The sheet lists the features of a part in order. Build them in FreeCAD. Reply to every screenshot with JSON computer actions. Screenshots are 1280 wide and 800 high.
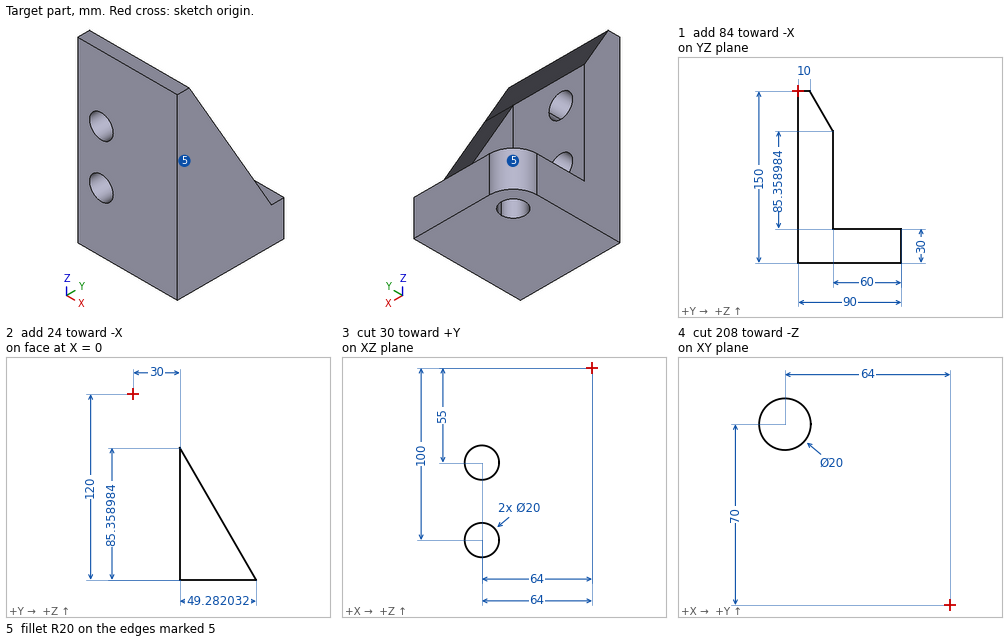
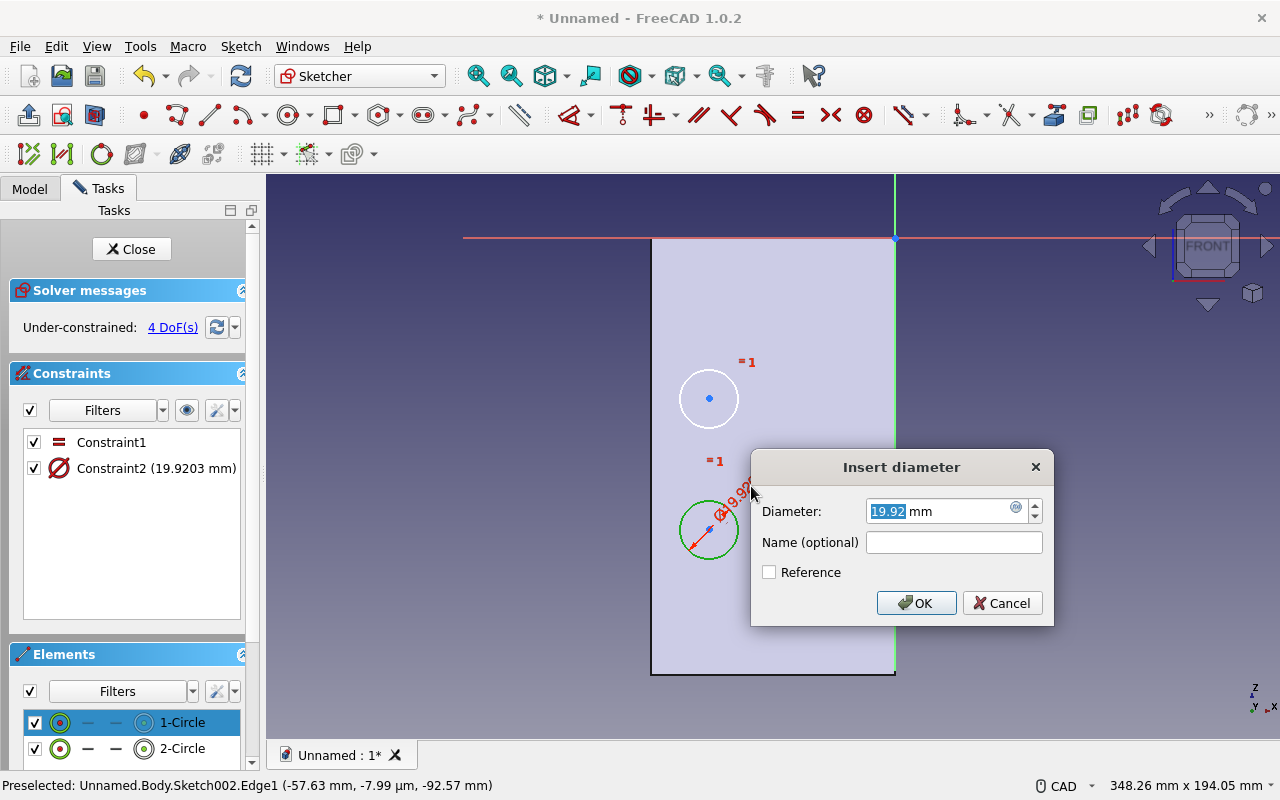
{"action": "type", "text": "20"}
{"action": "key", "text": "Return"}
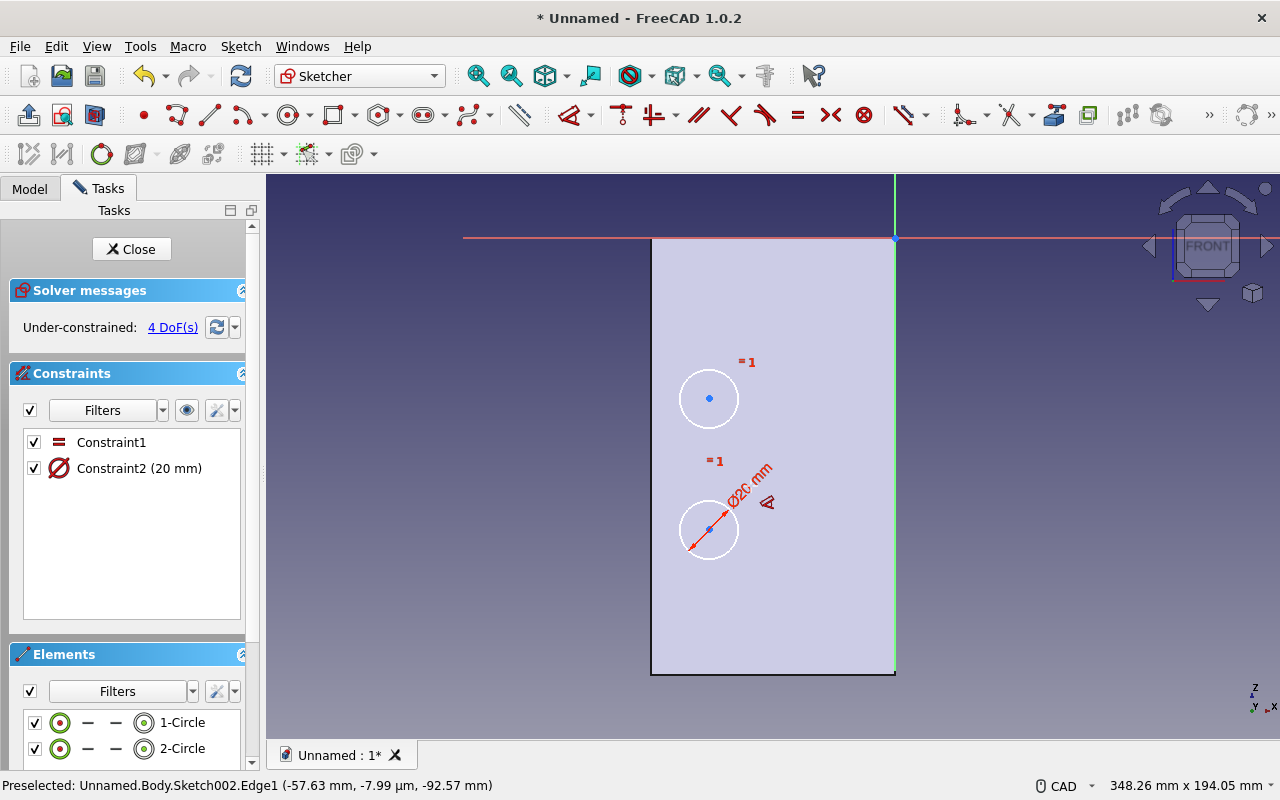
{"action": "left_click", "coordinate": [709, 530]}
{"action": "left_click", "coordinate": [802, 204]}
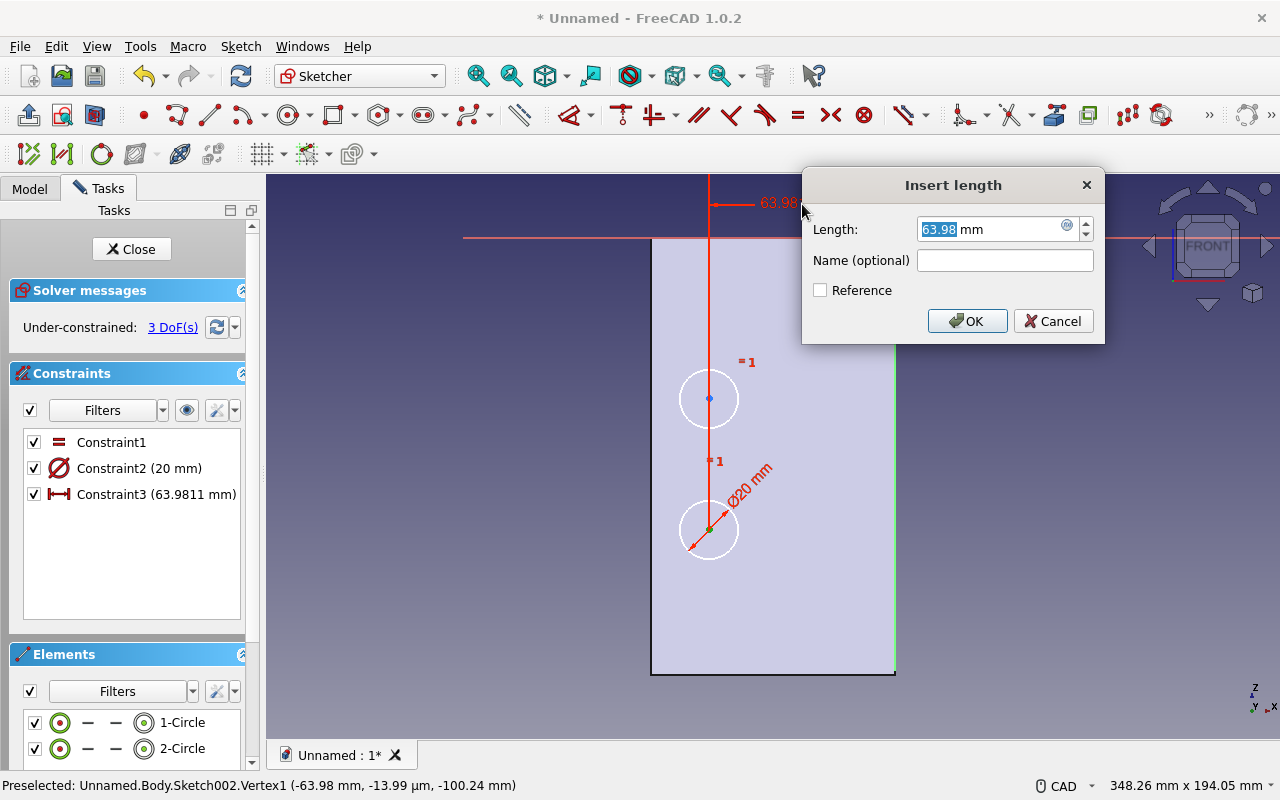
{"action": "type", "text": "64"}
{"action": "key", "text": "Return"}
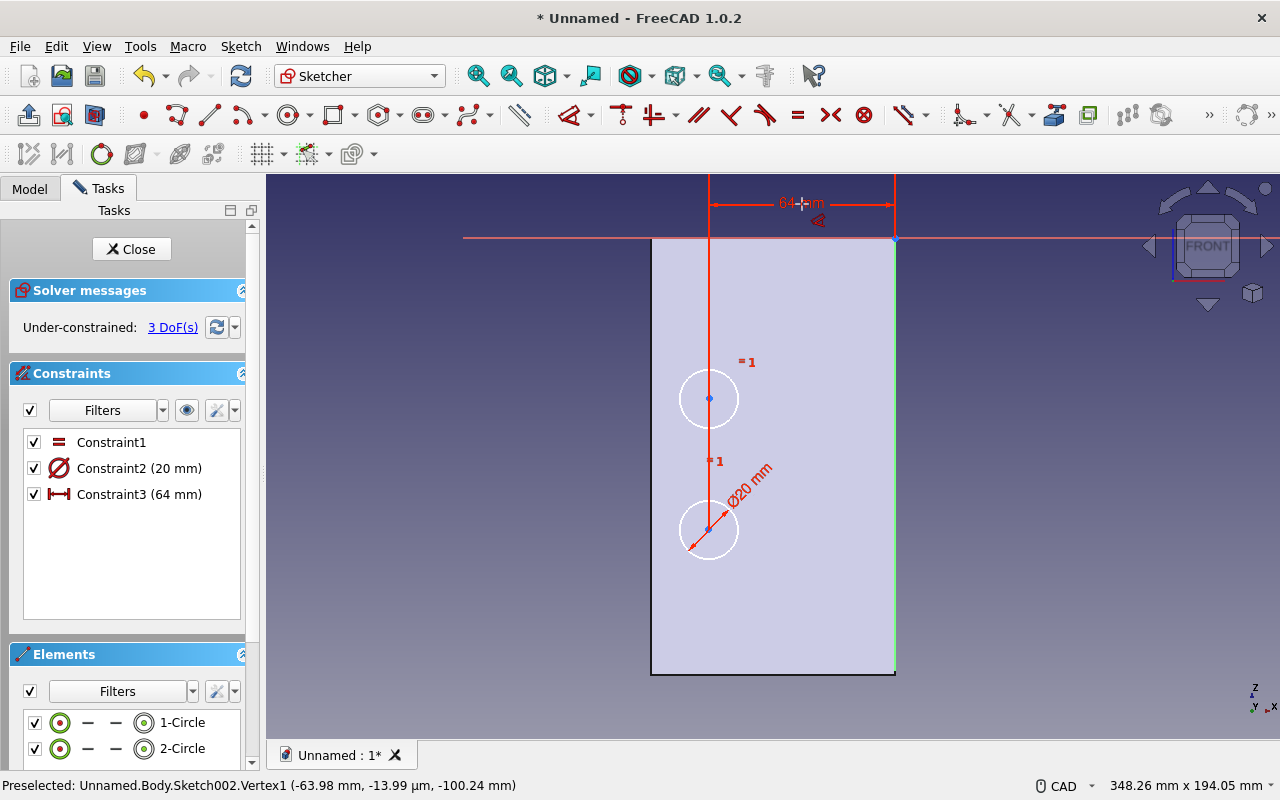
{"action": "left_click", "coordinate": [709, 399]}
{"action": "left_click", "coordinate": [802, 433]}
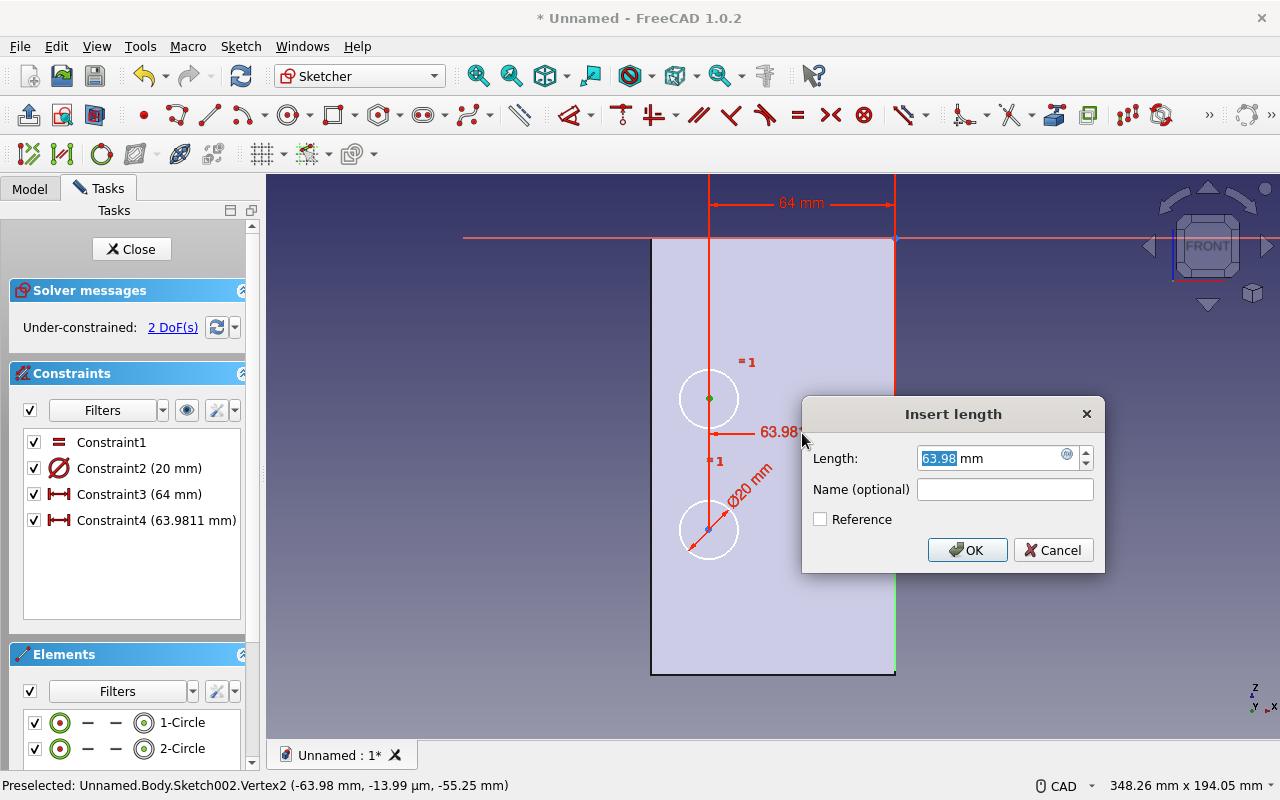
{"action": "type", "text": "64"}
{"action": "key", "text": "Return"}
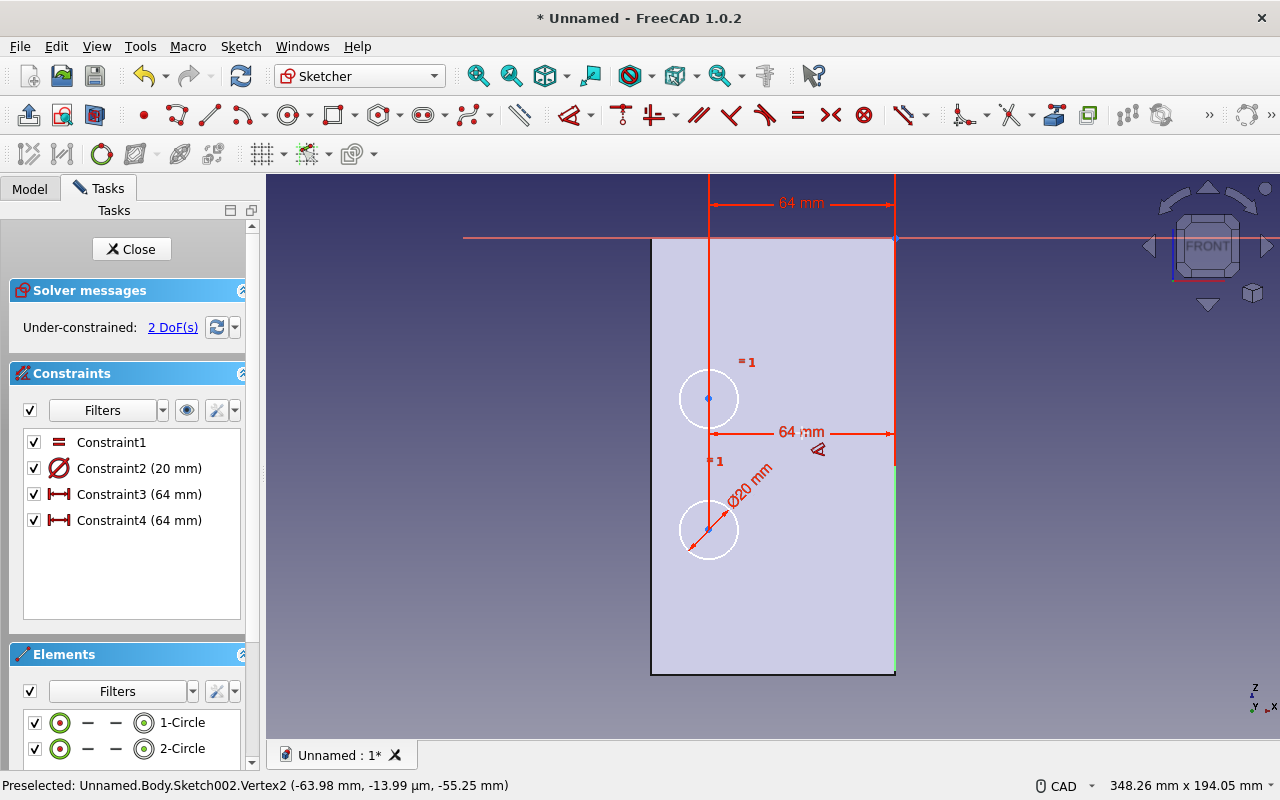
{"action": "left_click", "coordinate": [709, 399]}
{"action": "left_click", "coordinate": [929, 319]}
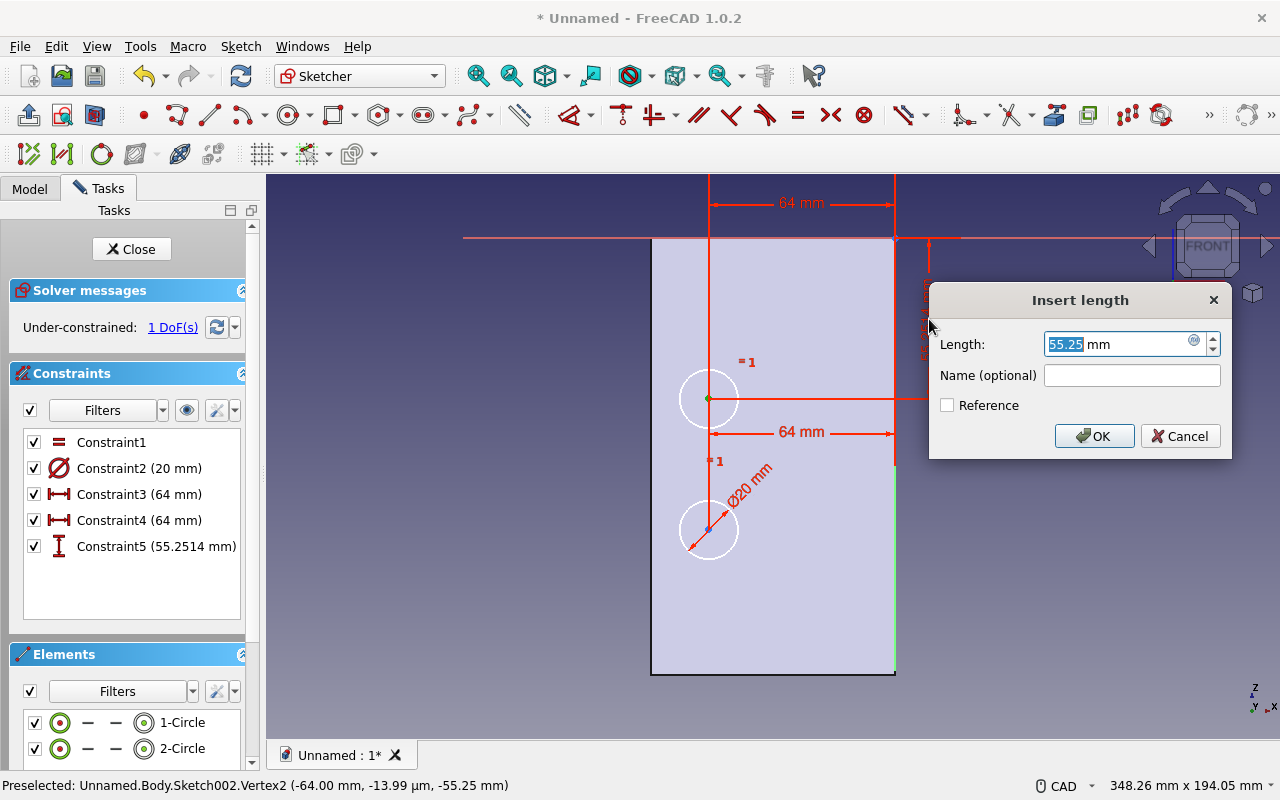
{"action": "type", "text": "55"}
{"action": "key", "text": "Return"}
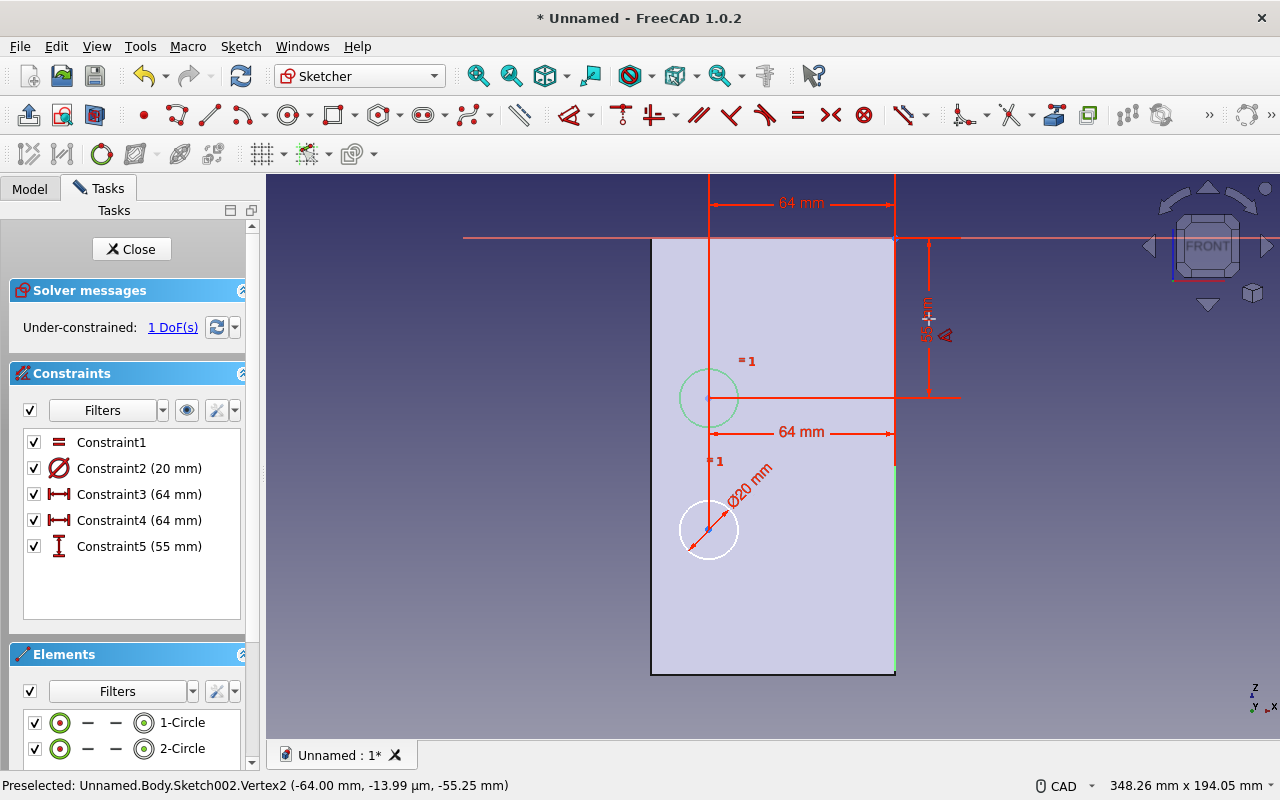
{"action": "left_click", "coordinate": [709, 530]}
{"action": "left_click", "coordinate": [929, 384]}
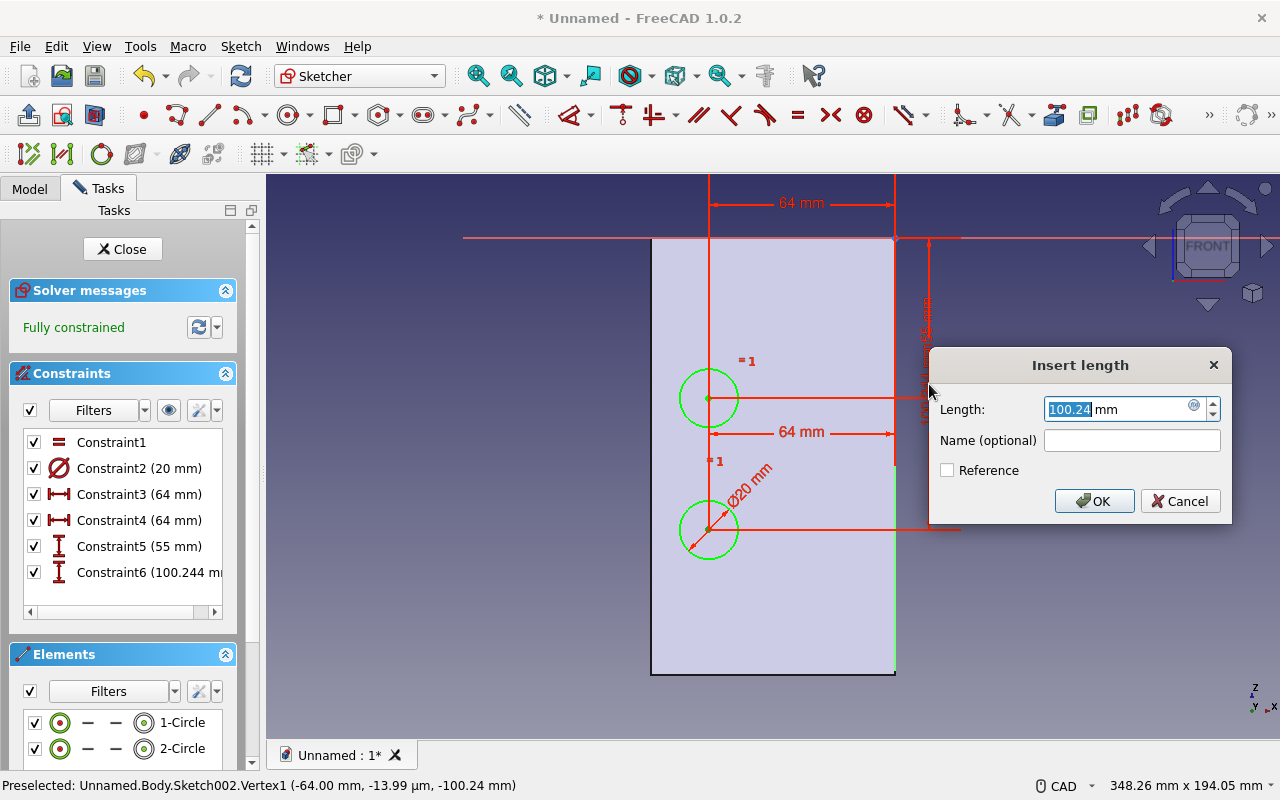
{"action": "type", "text": "100"}
{"action": "key", "text": "Return"}
{"action": "key", "text": "Escape"}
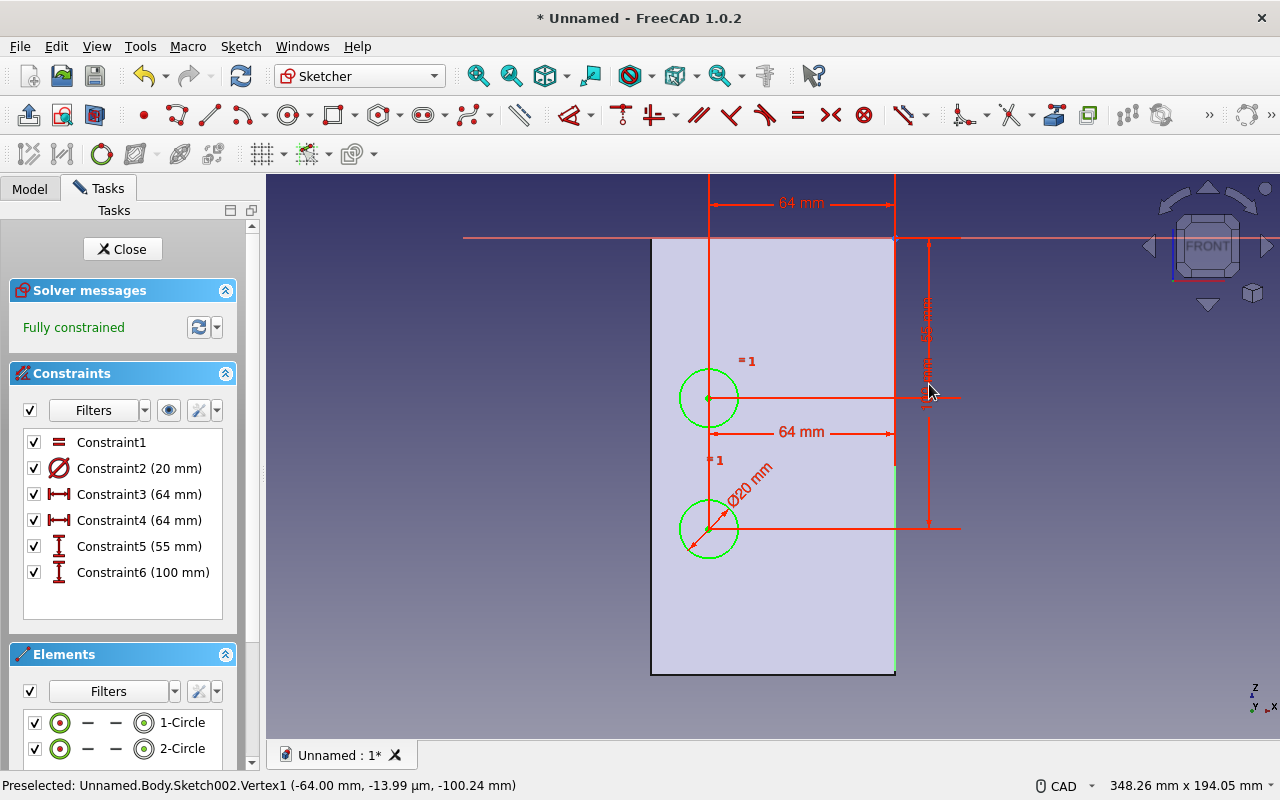
{"action": "left_click", "coordinate": [123, 249]}